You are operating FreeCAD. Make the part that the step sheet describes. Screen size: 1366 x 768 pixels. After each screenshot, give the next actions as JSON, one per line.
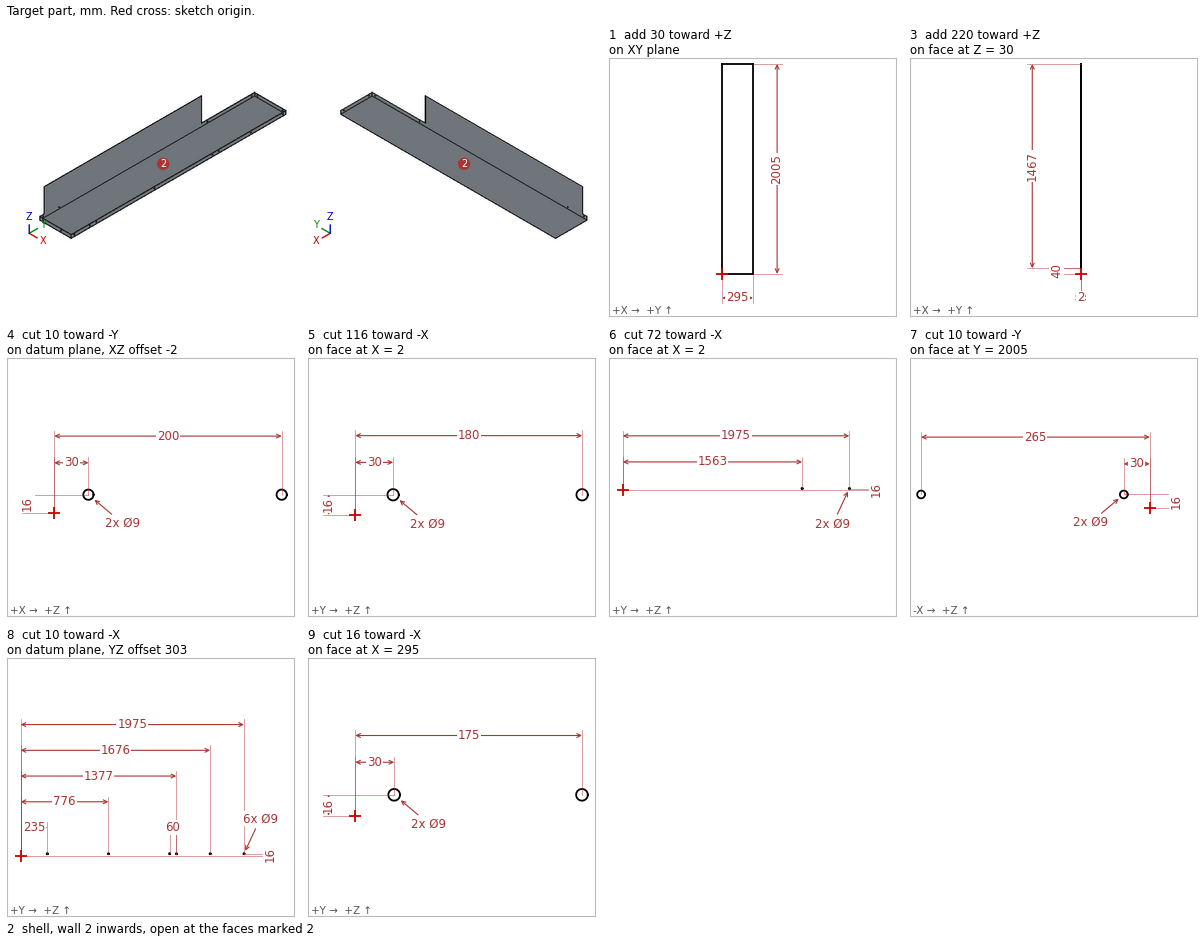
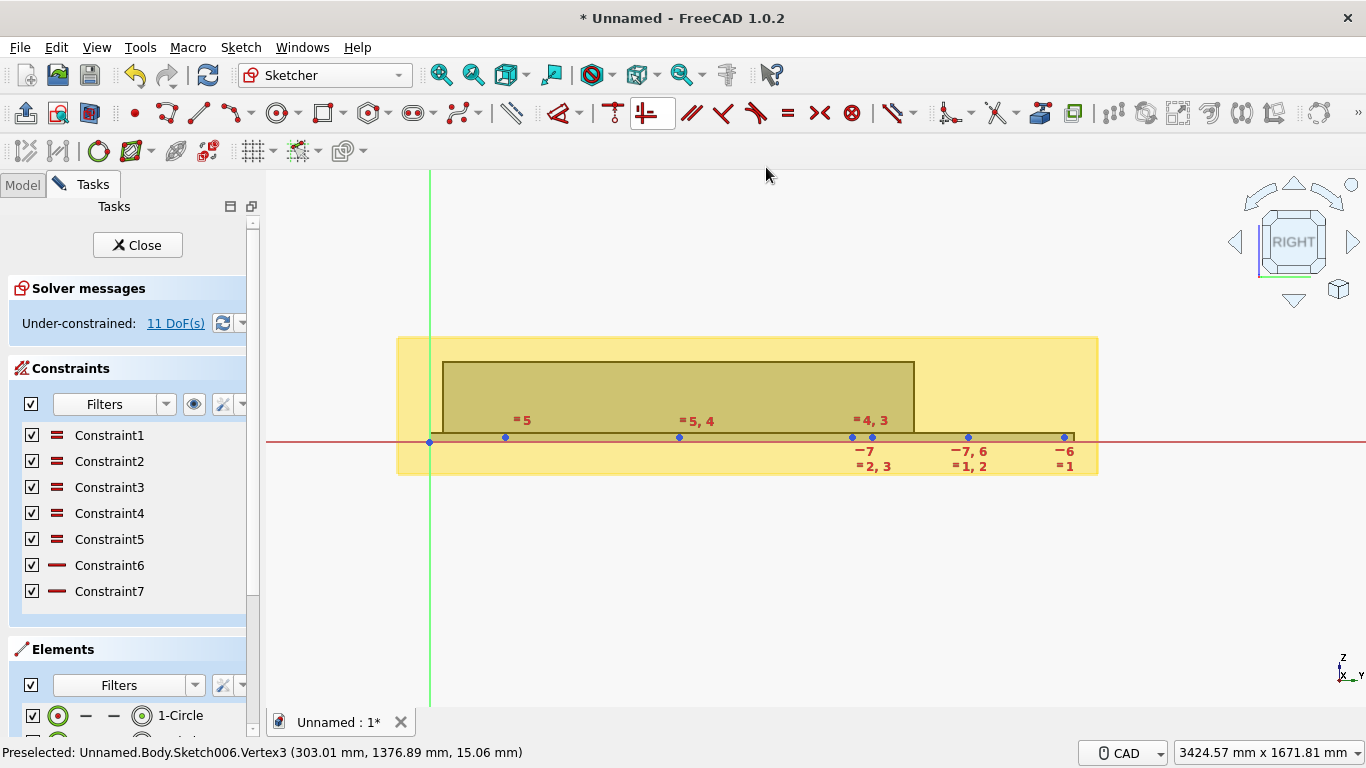
{"action": "left_click", "coordinate": [872, 437]}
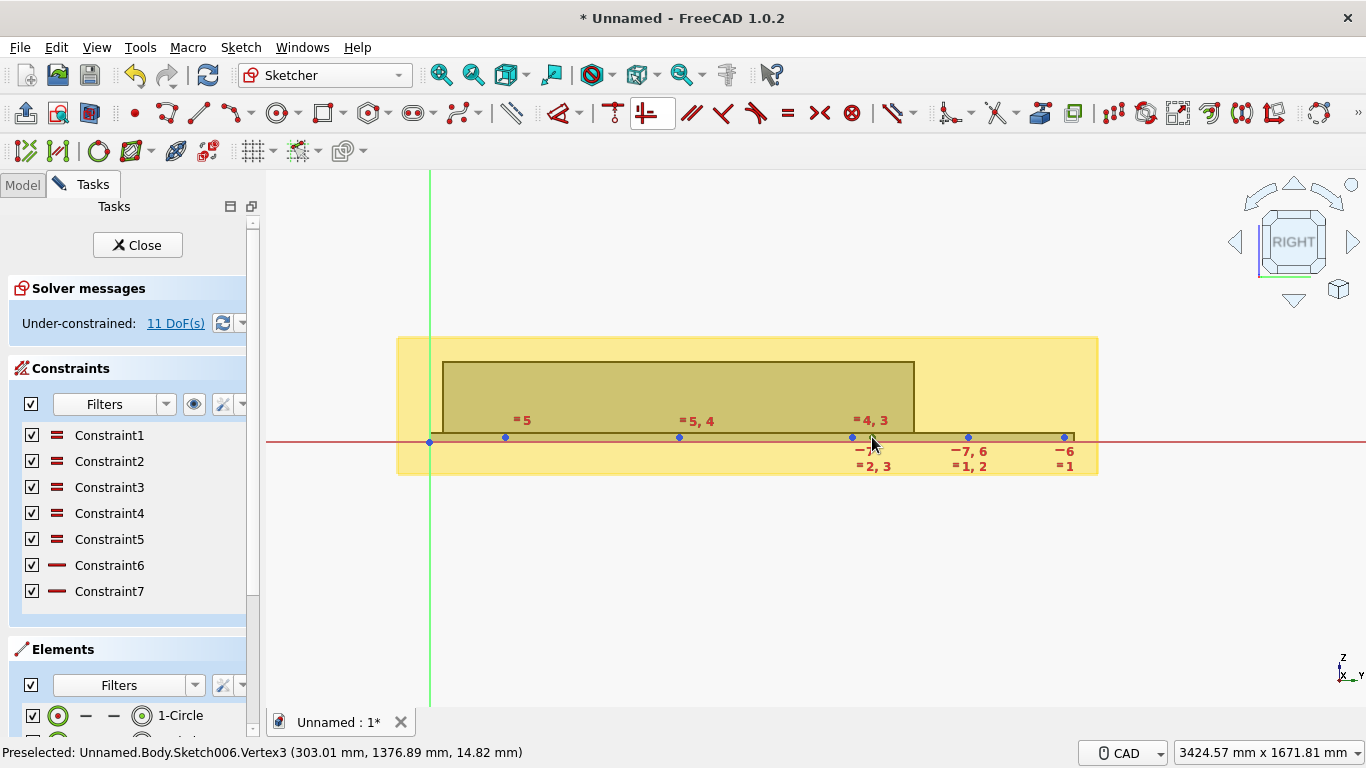
{"action": "left_click", "coordinate": [853, 437]}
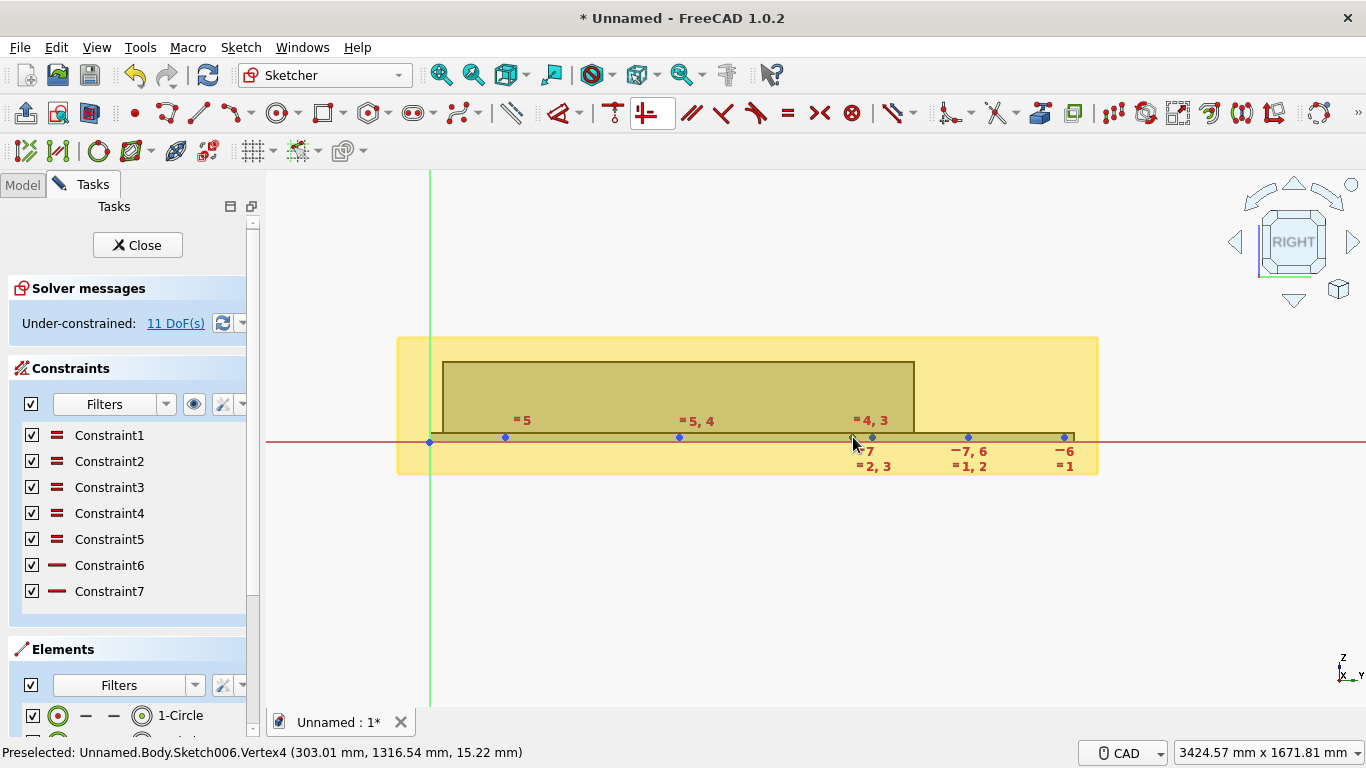
{"action": "key", "text": "h"}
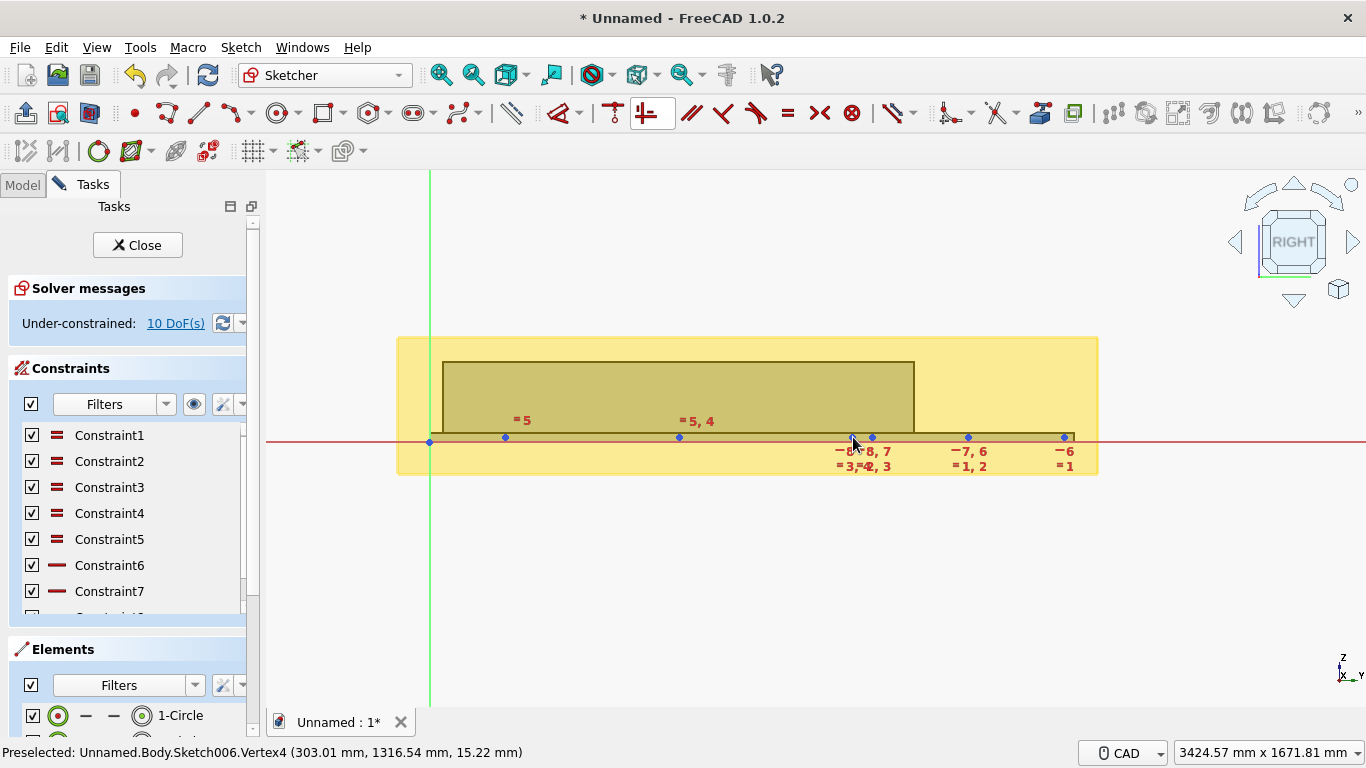
{"action": "left_click", "coordinate": [853, 437]}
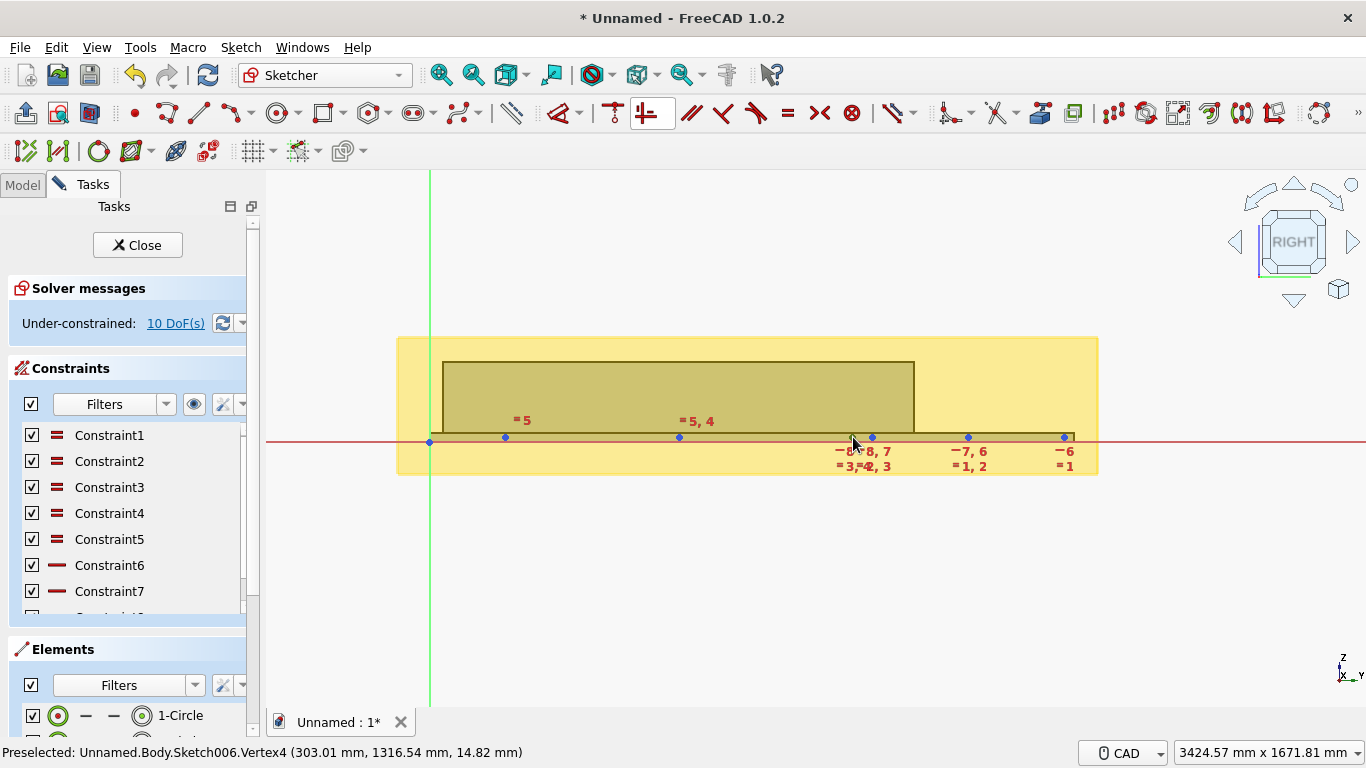
{"action": "left_click", "coordinate": [679, 437]}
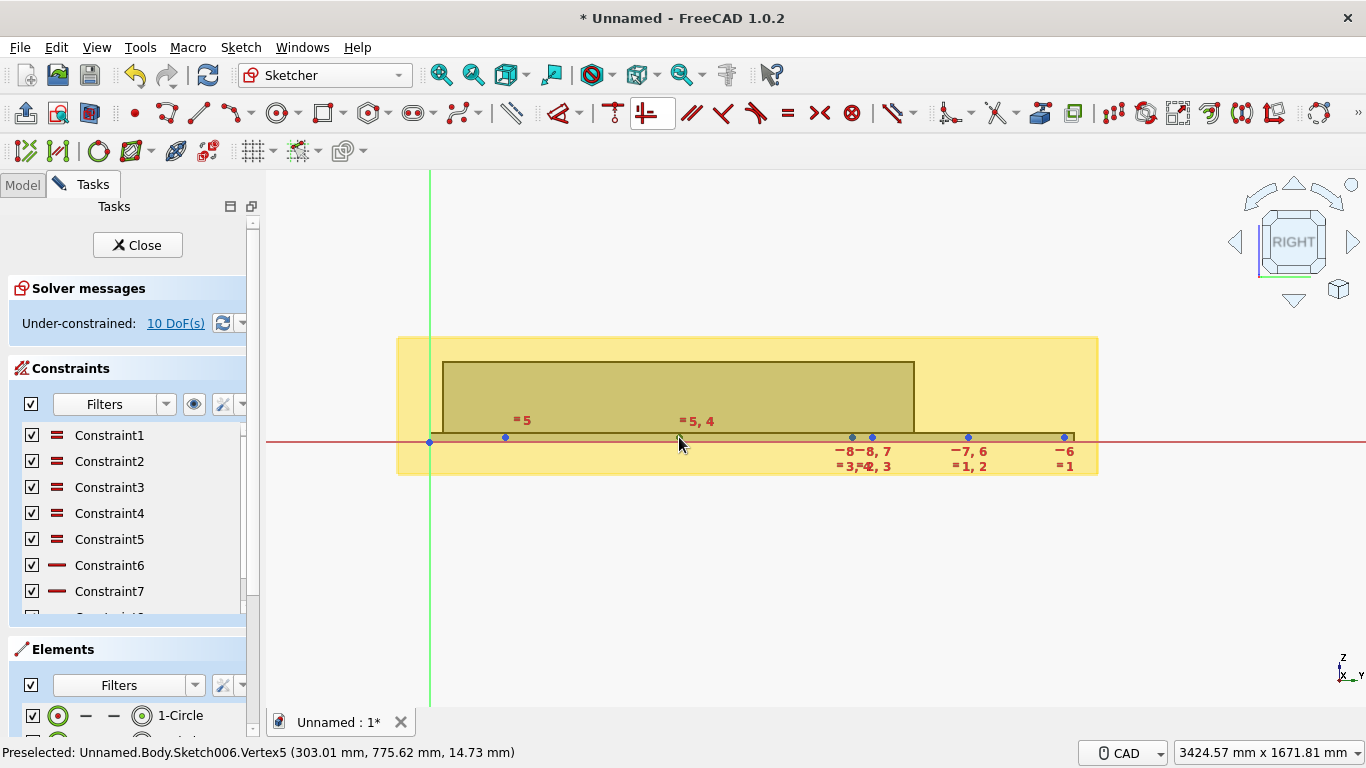
{"action": "left_click", "coordinate": [670, 114]}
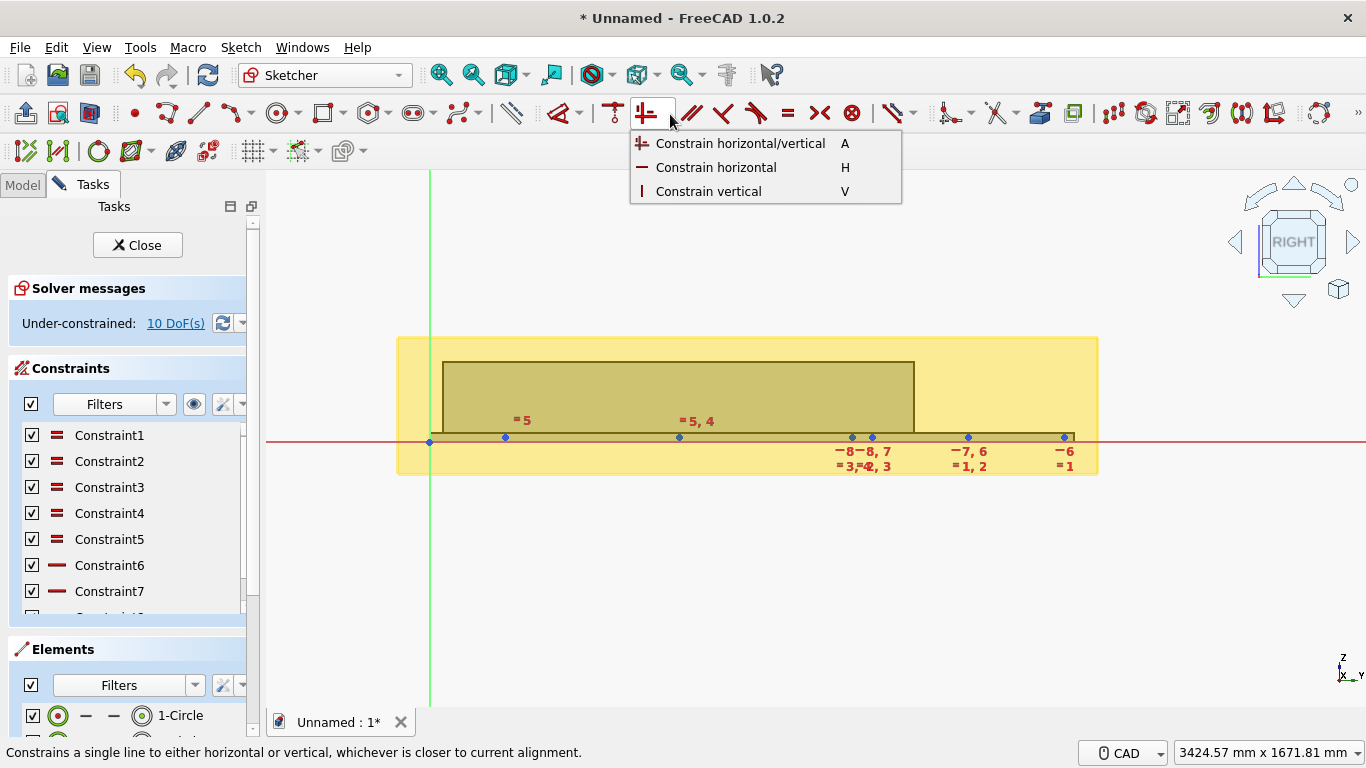
{"action": "left_click", "coordinate": [766, 167]}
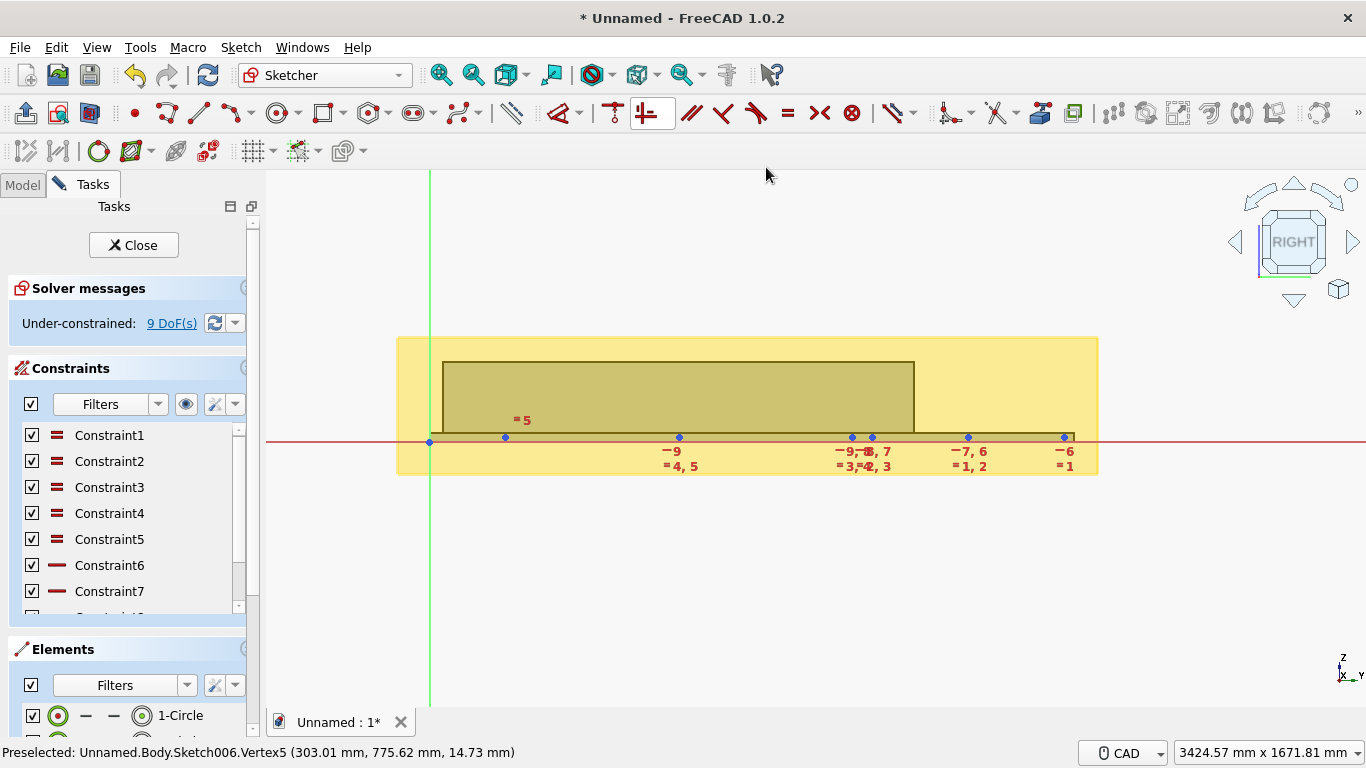
{"action": "left_click", "coordinate": [679, 437]}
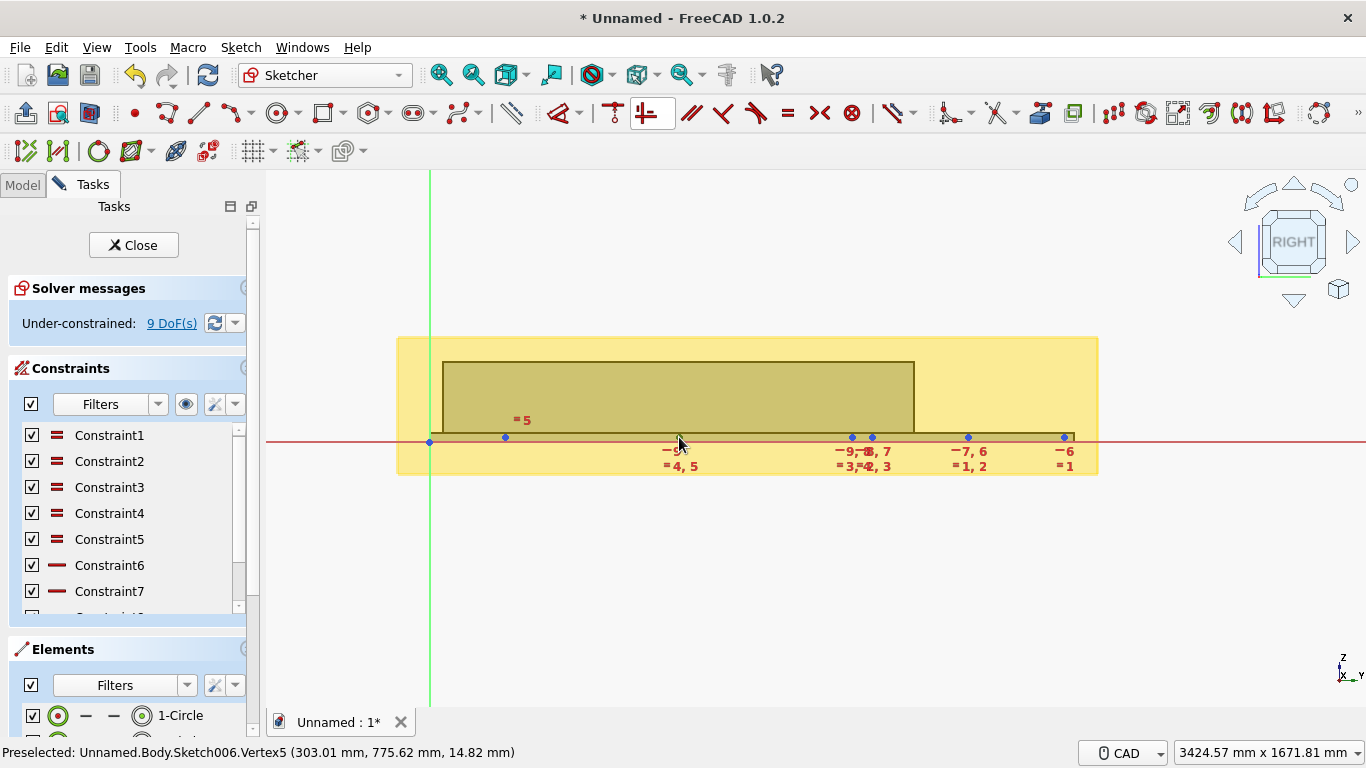
{"action": "left_click", "coordinate": [505, 437]}